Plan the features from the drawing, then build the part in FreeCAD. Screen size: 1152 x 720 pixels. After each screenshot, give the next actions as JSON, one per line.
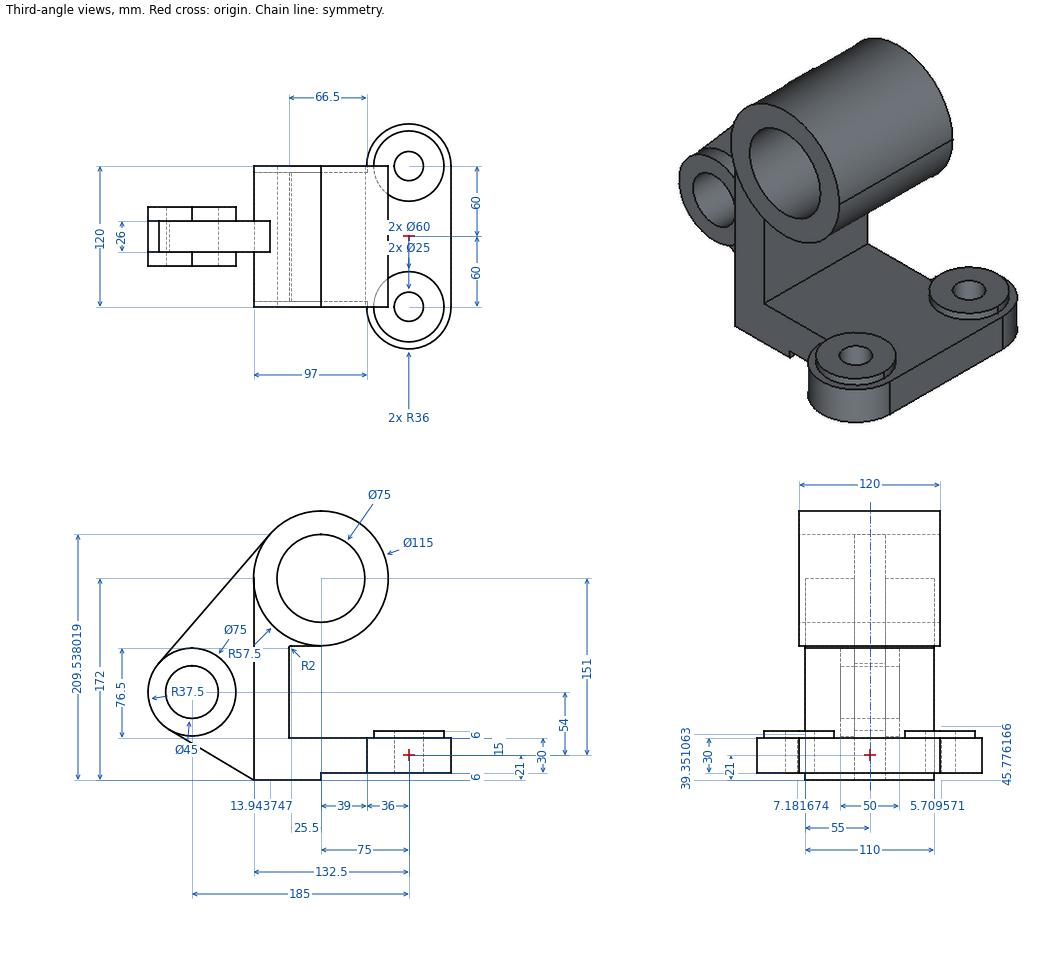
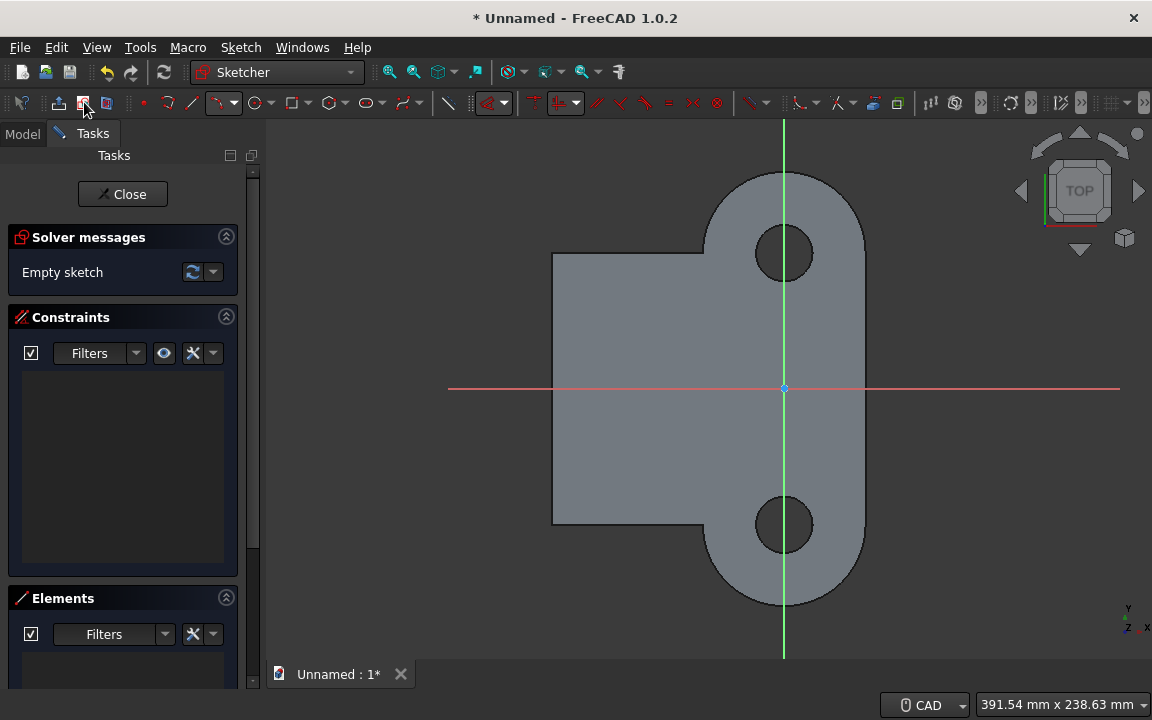
{"action": "key", "text": "g c"}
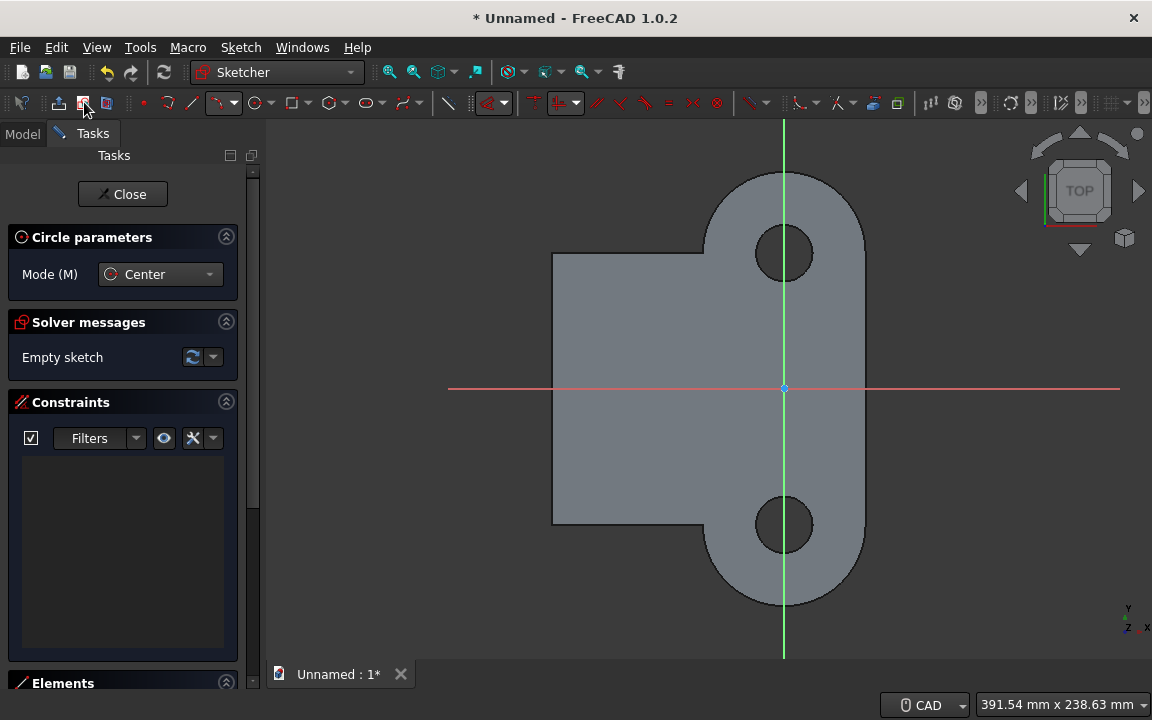
{"action": "left_click", "coordinate": [784, 525]}
{"action": "left_click", "coordinate": [832, 477]}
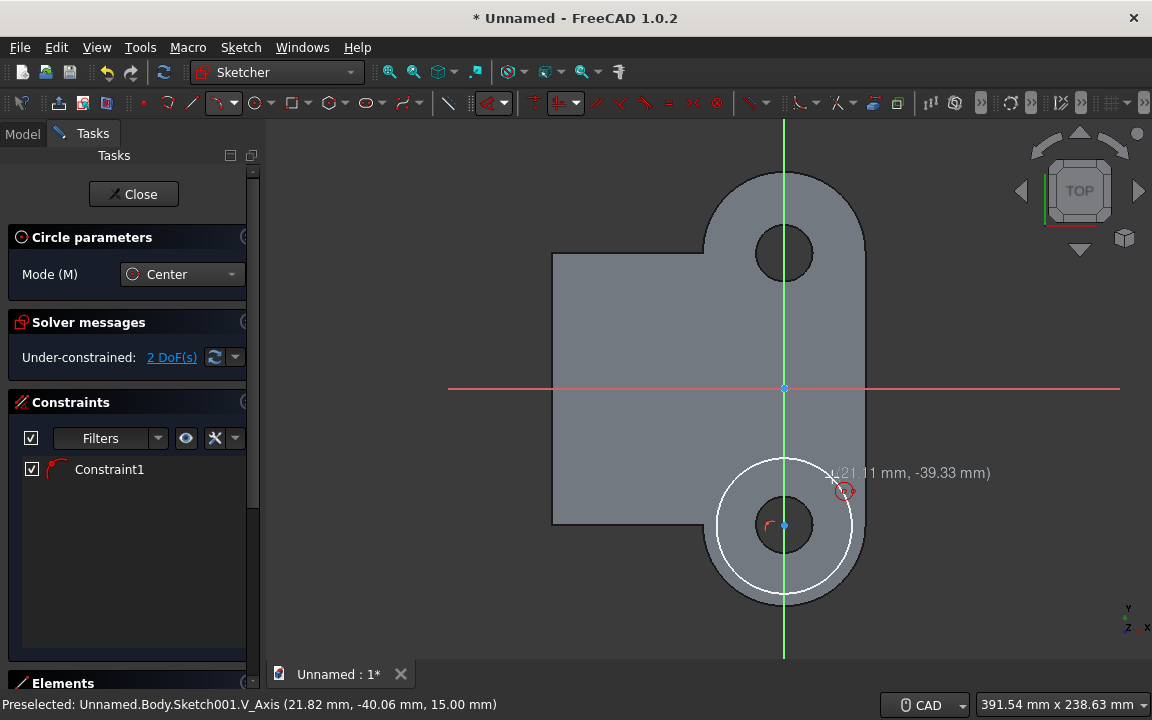
{"action": "left_click", "coordinate": [784, 253]}
{"action": "left_click", "coordinate": [832, 205]}
{"action": "key", "text": "Escape"}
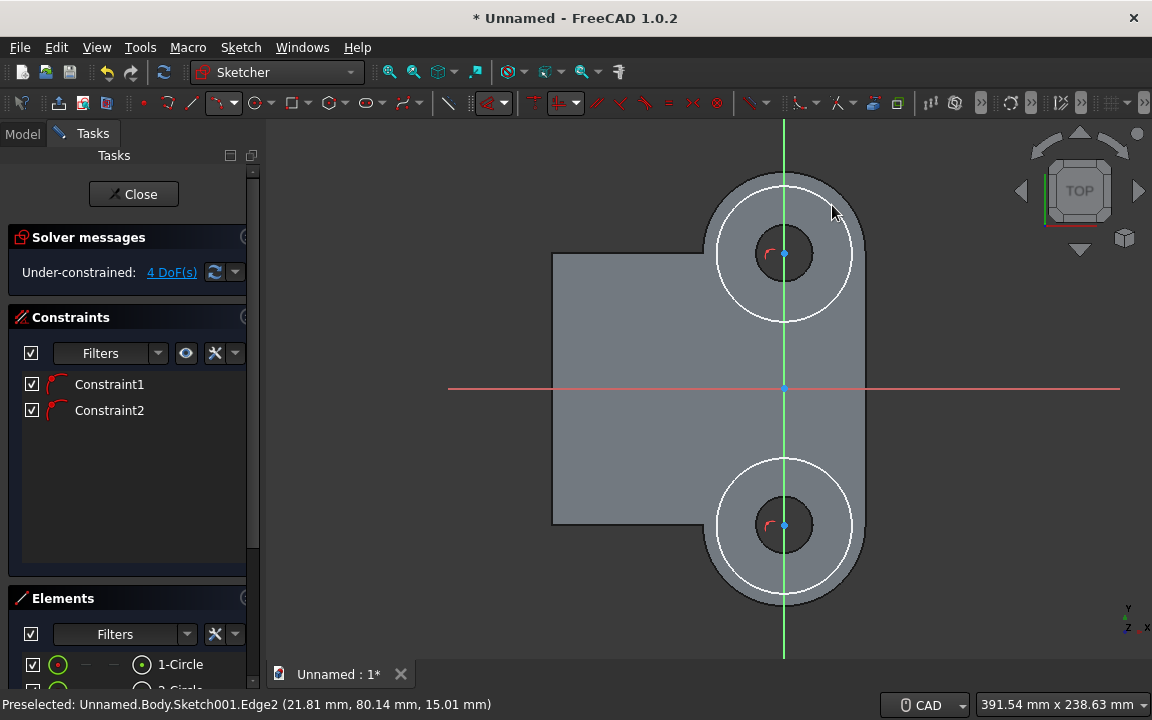
{"action": "left_click", "coordinate": [832, 478]}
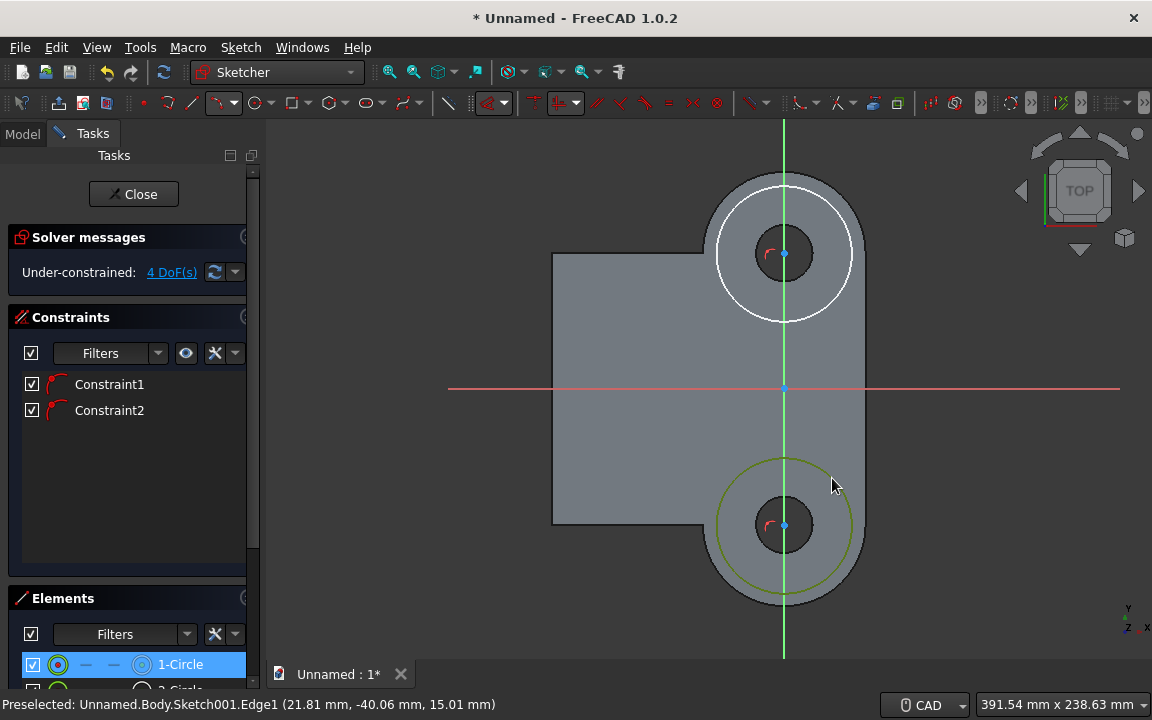
{"action": "left_click", "coordinate": [832, 206]}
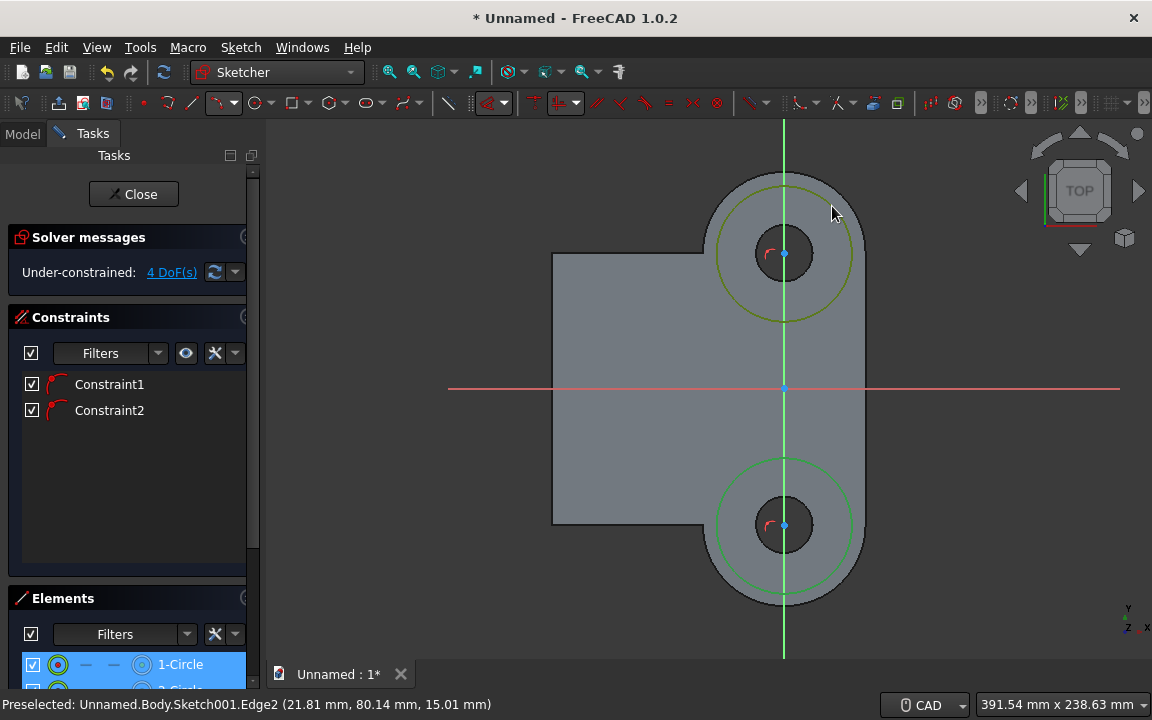
{"action": "key", "text": "e"}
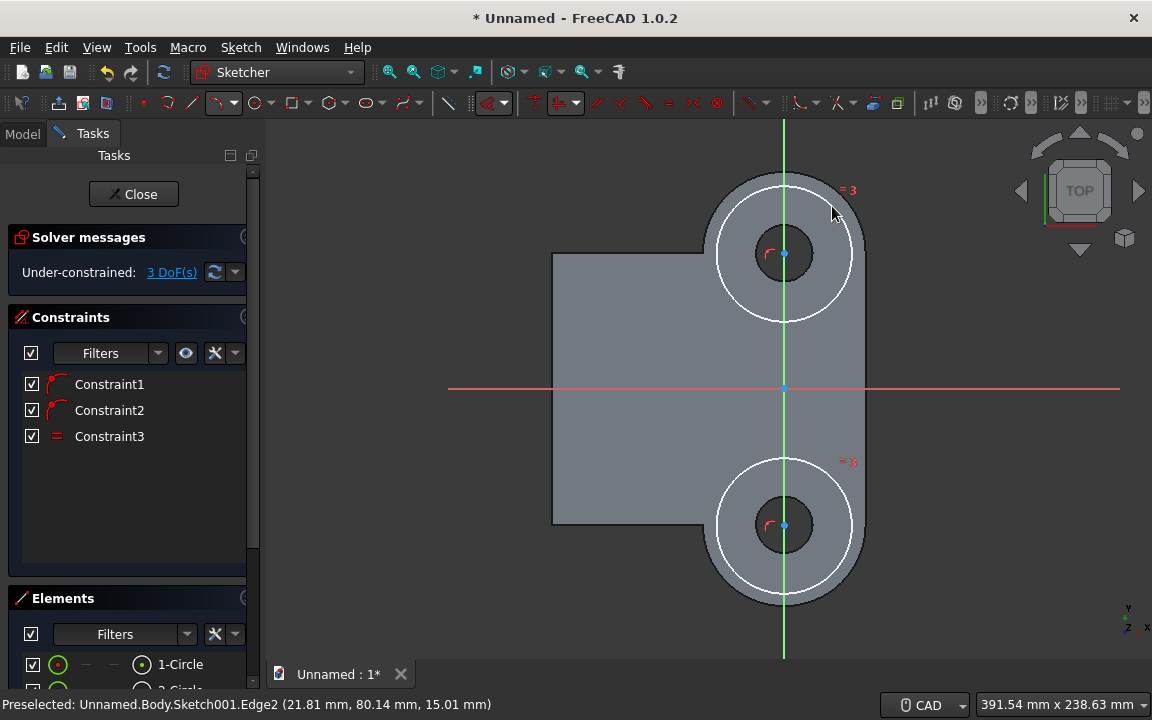
{"action": "left_click", "coordinate": [832, 478]}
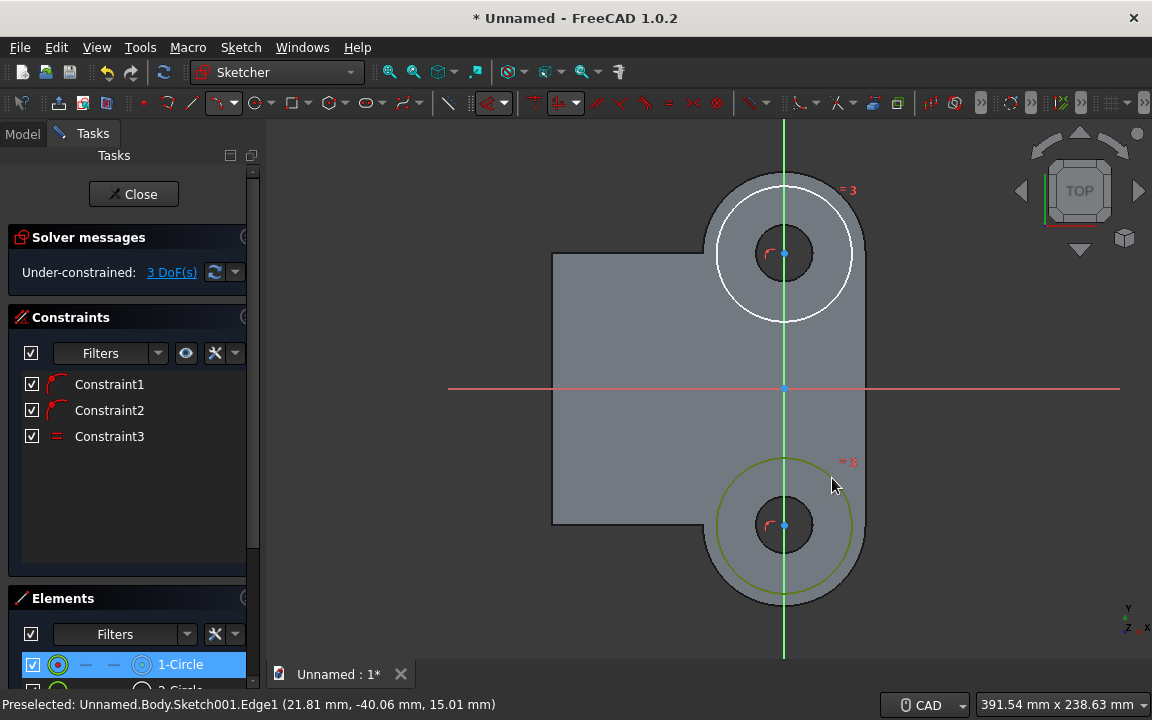
{"action": "key", "text": "k o"}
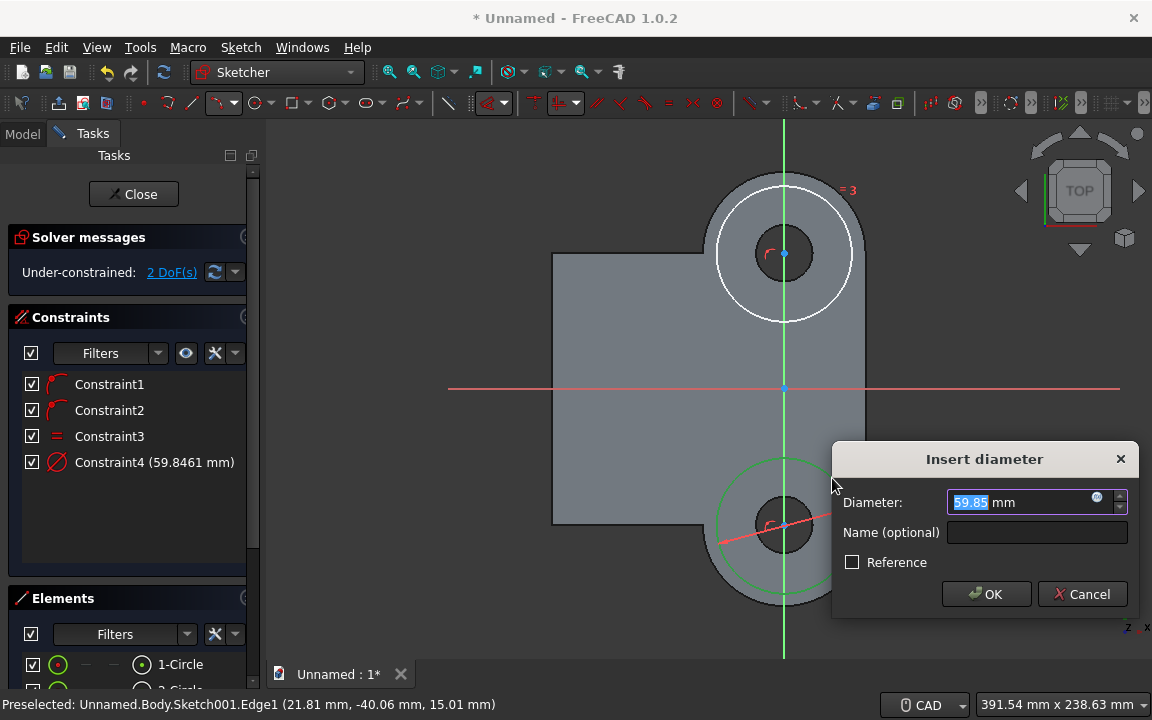
{"action": "type", "text": "60"}
{"action": "key", "text": "Return"}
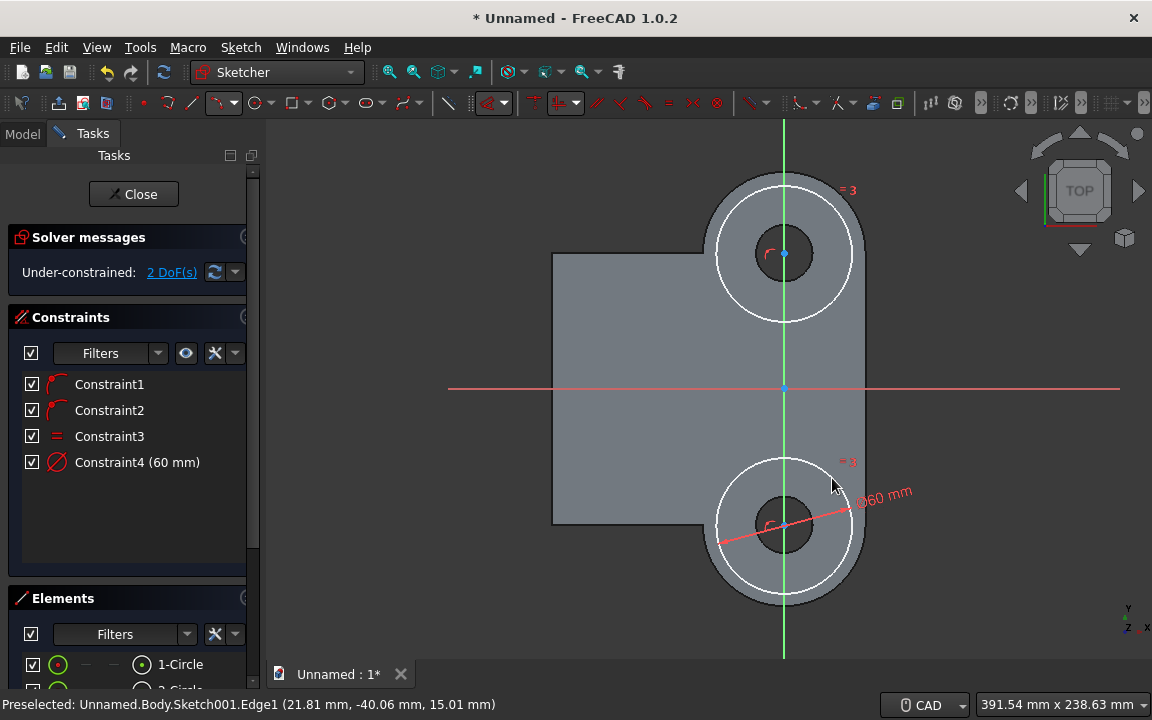
{"action": "left_click", "coordinate": [784, 526]}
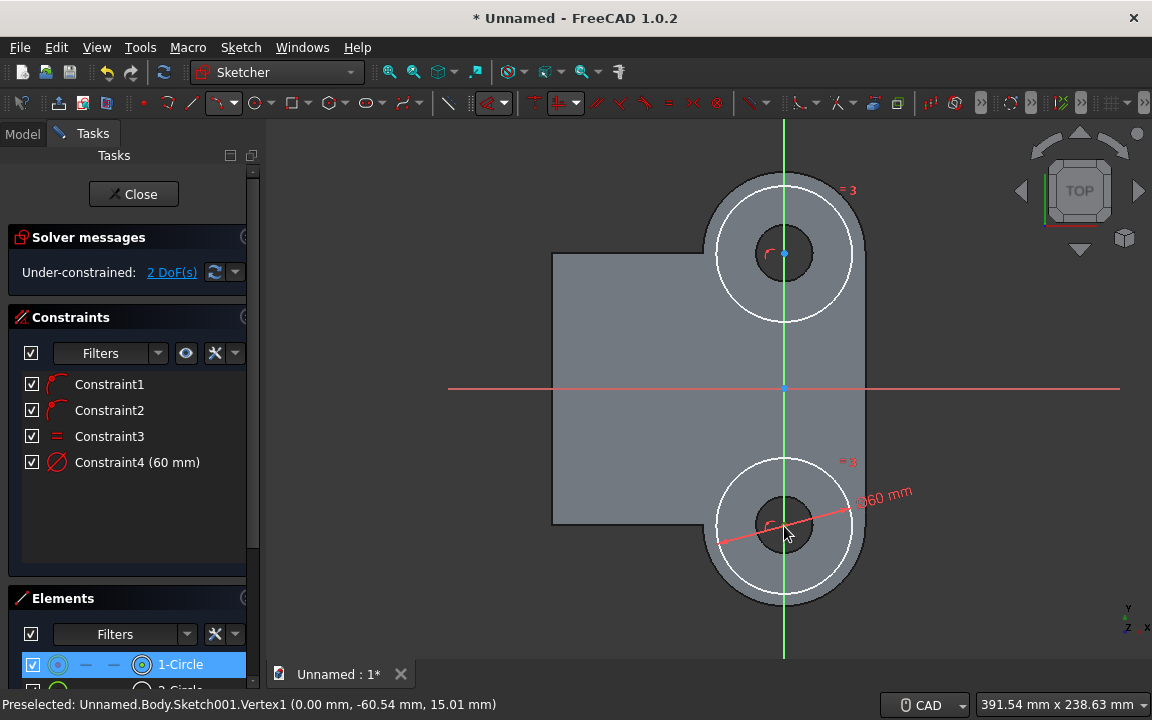
{"action": "key", "text": "i"}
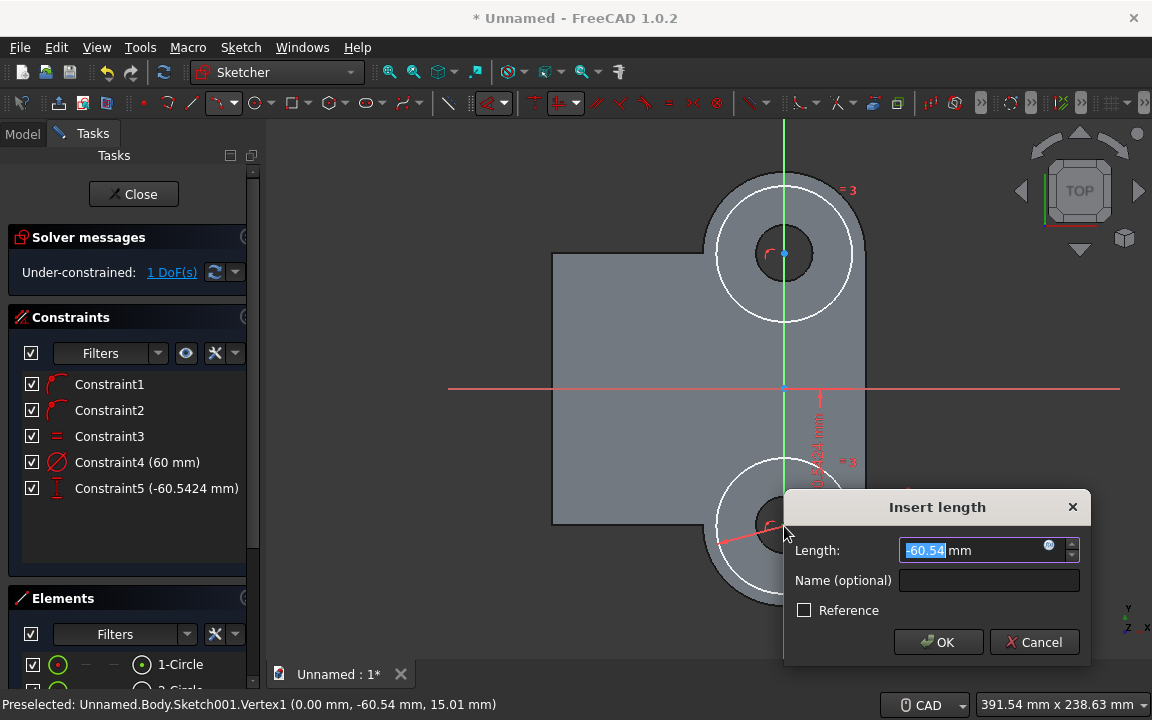
{"action": "type", "text": "-60"}
{"action": "key", "text": "Return"}